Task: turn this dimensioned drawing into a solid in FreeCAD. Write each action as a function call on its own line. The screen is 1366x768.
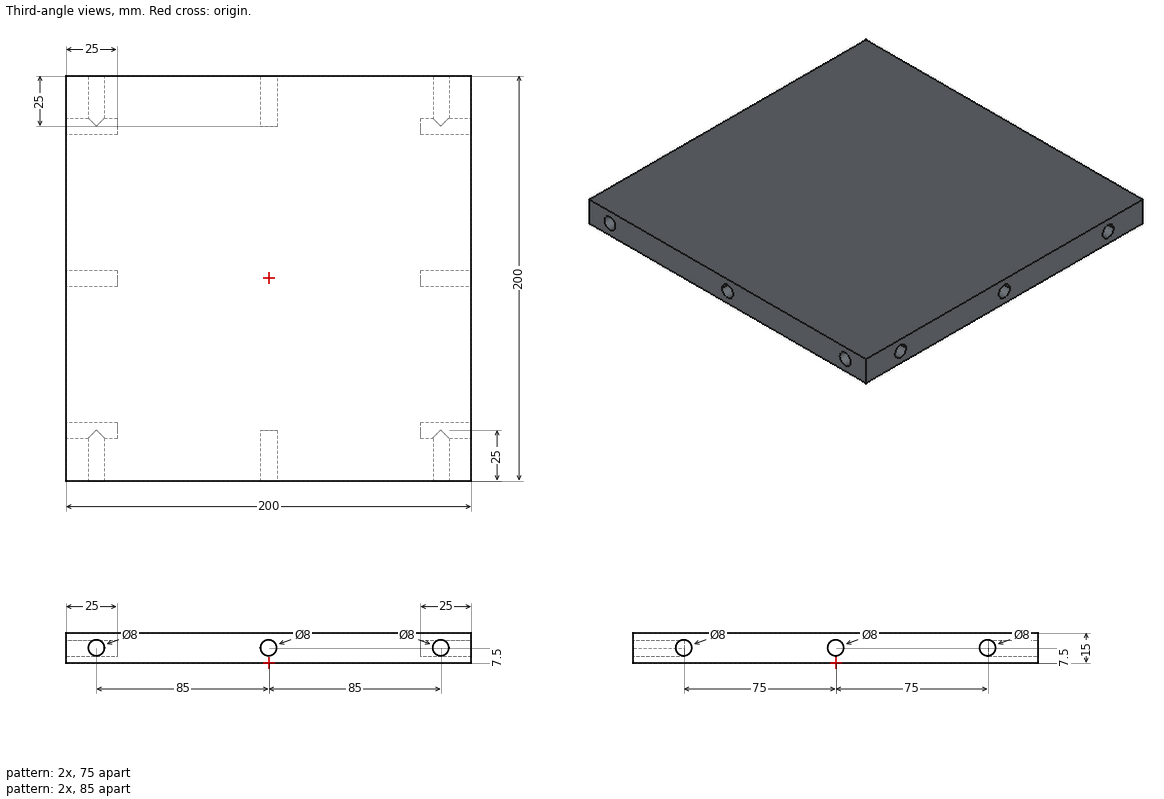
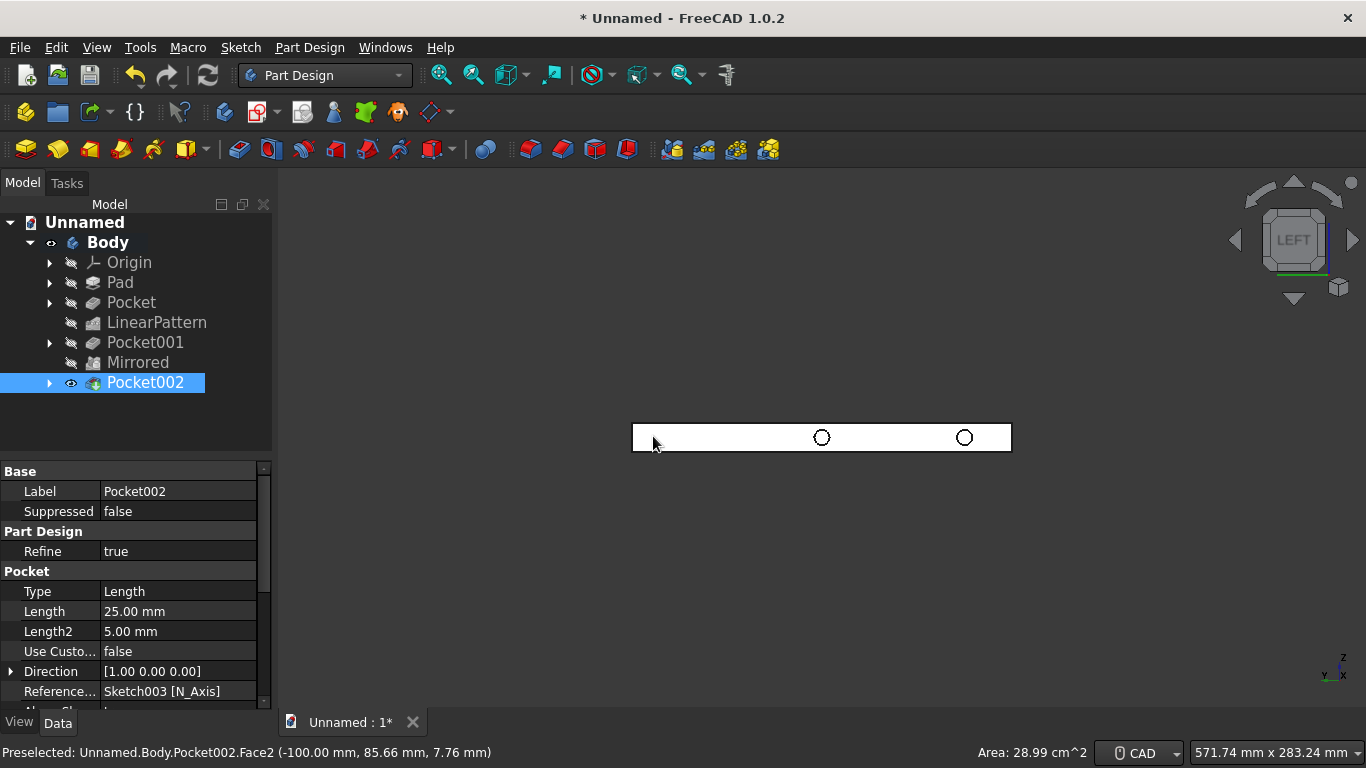
click(258, 112)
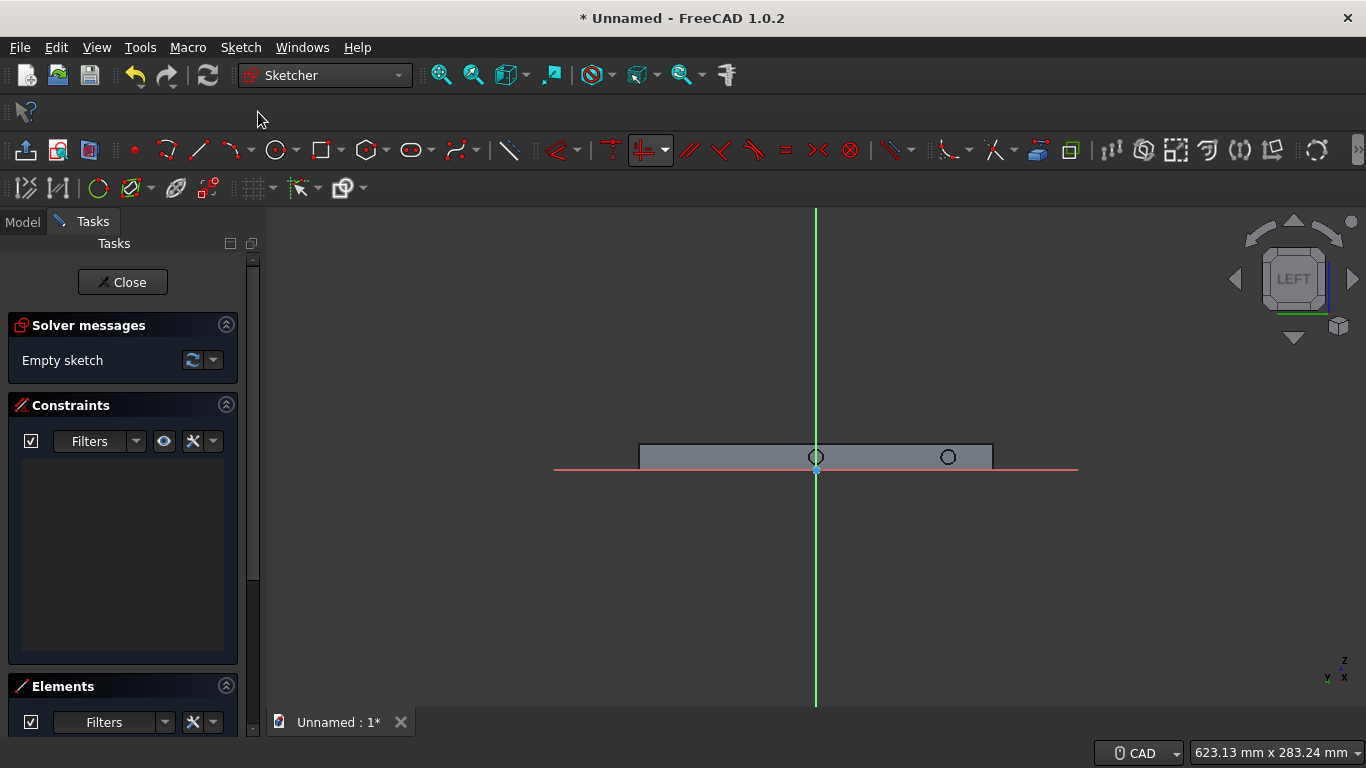
scroll(680, 457, up, 15)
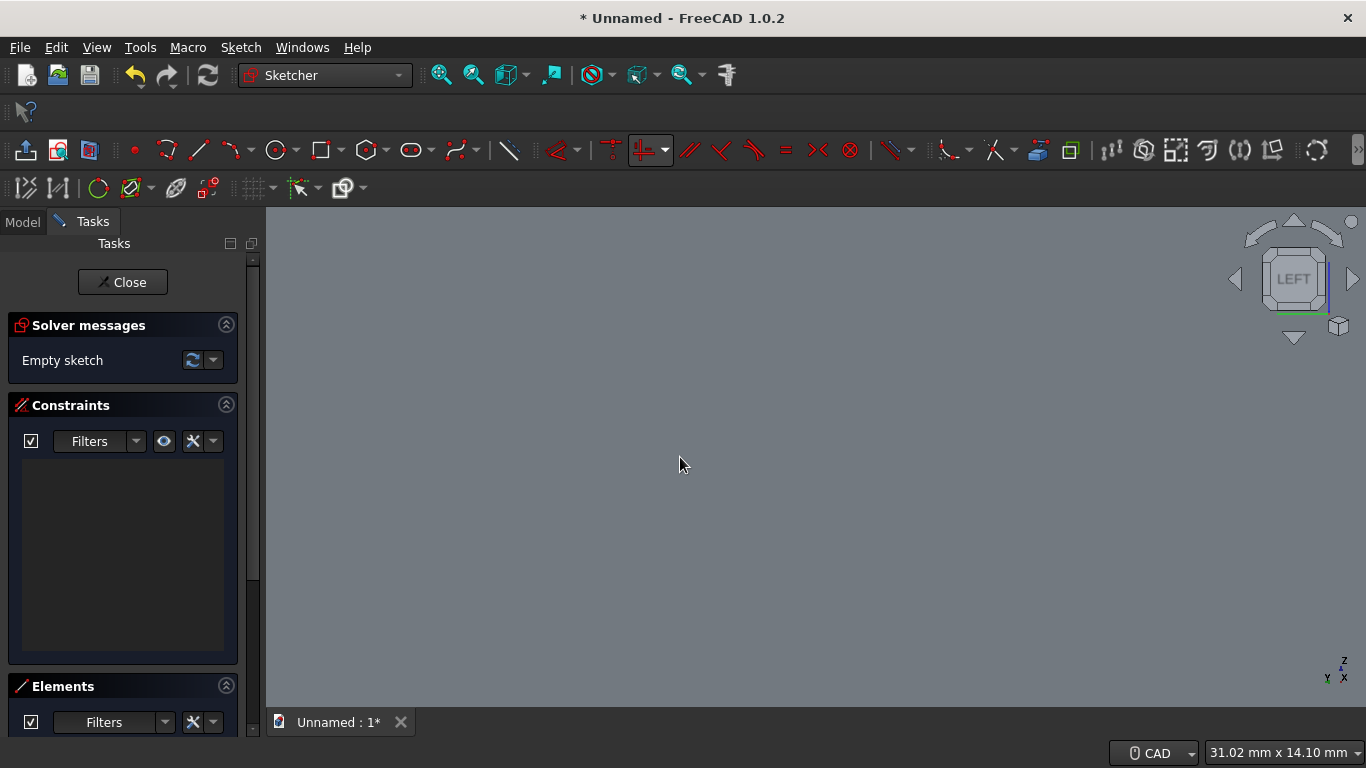
click(276, 150)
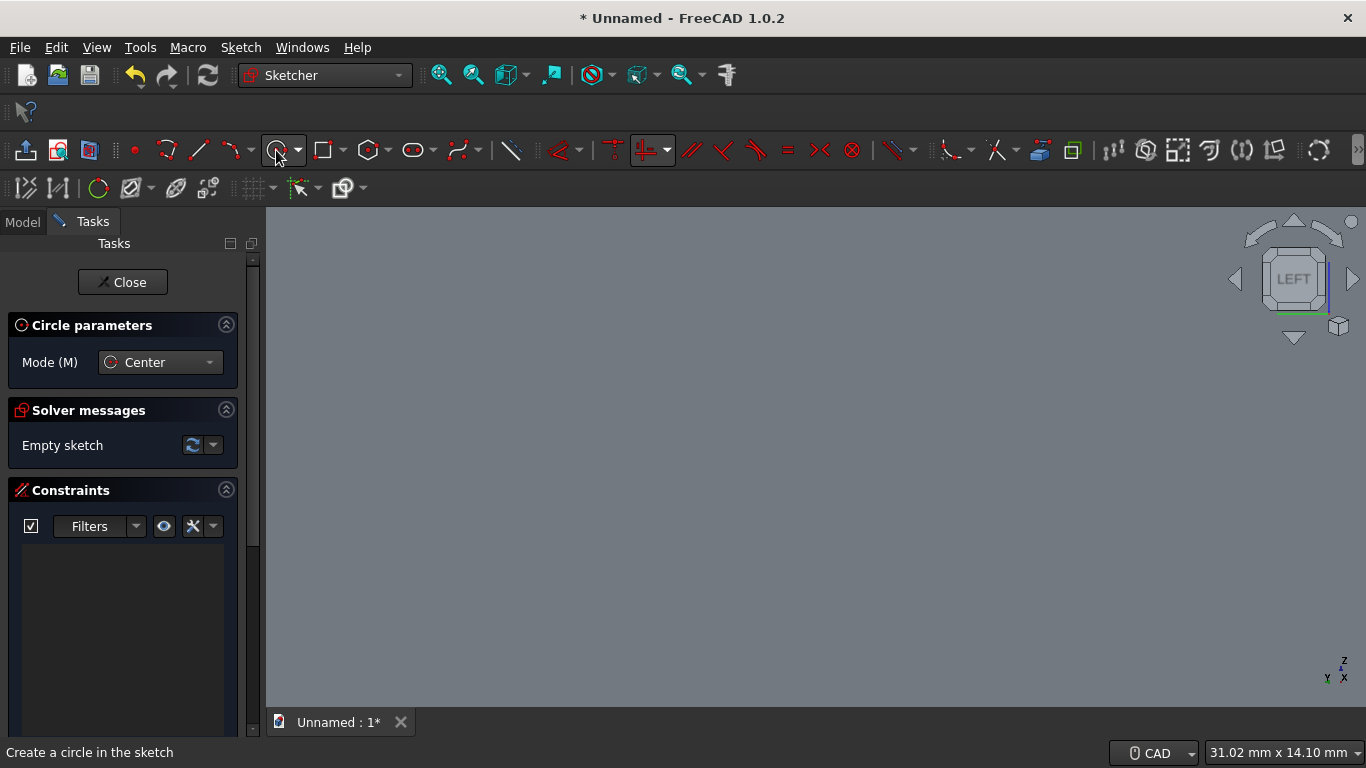
click(745, 447)
move(845, 347)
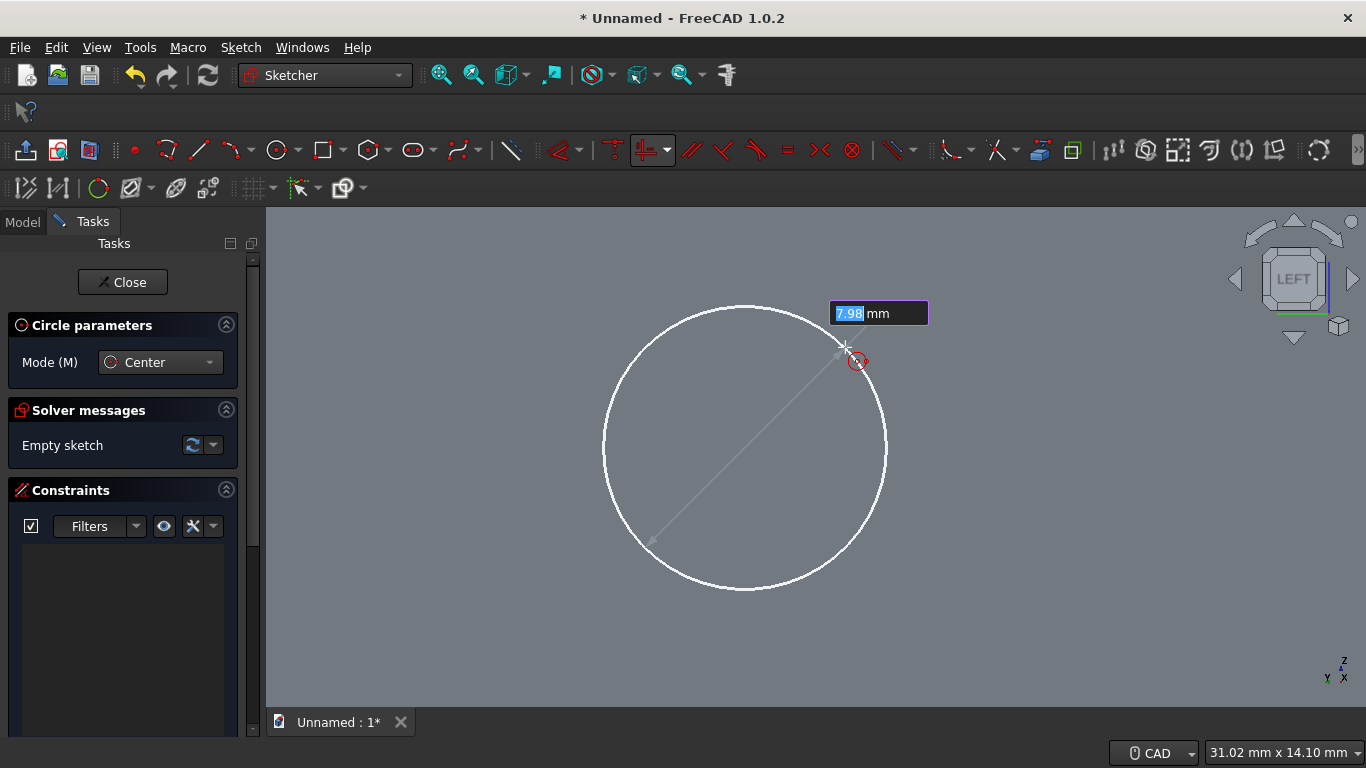
text(8)
key(Return)
key(Escape)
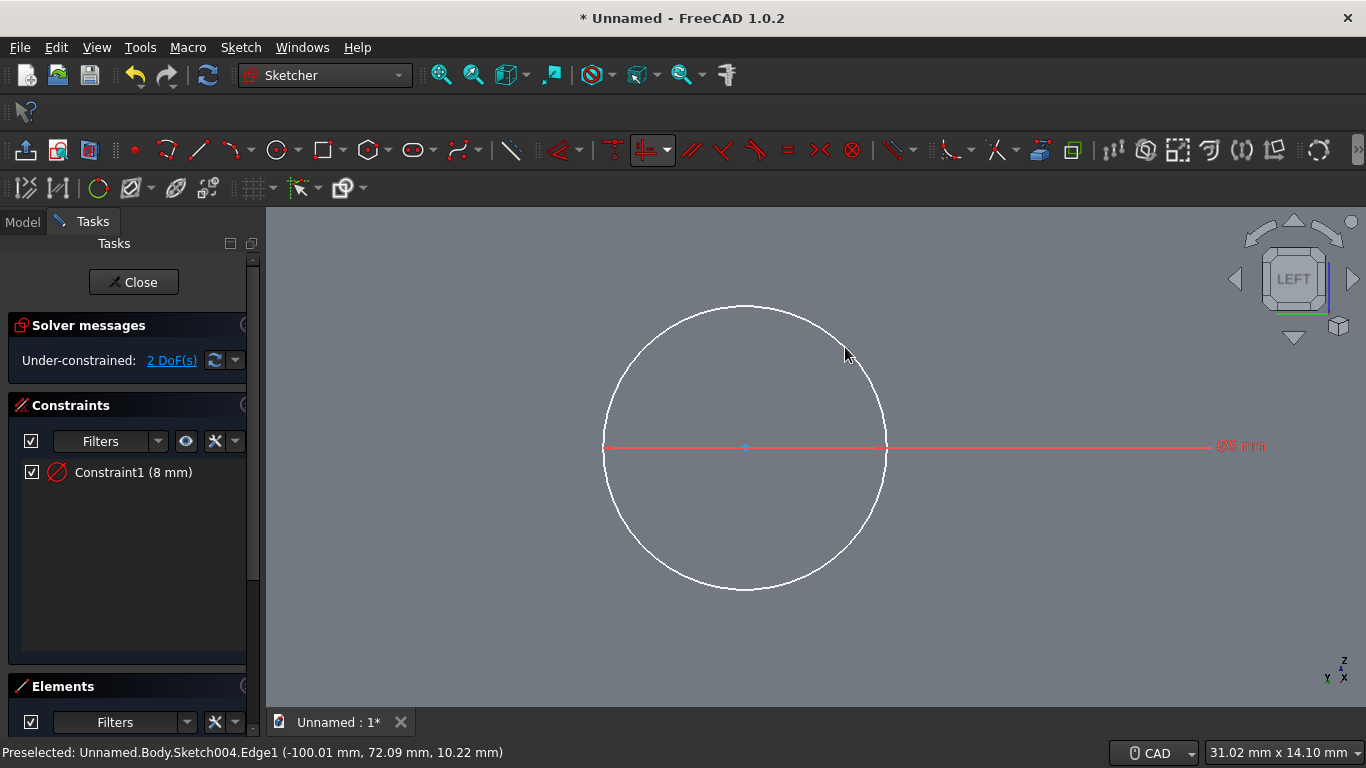
key(d)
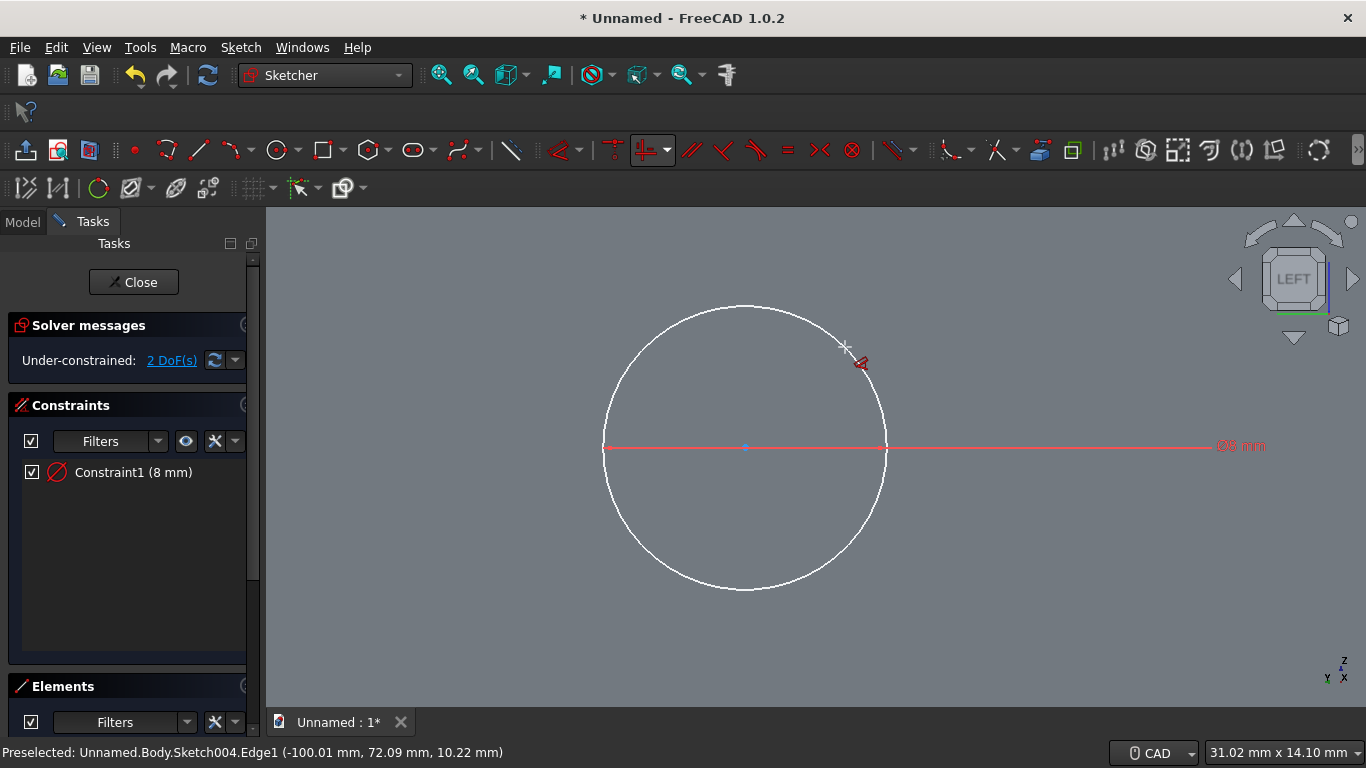
click(745, 448)
click(973, 414)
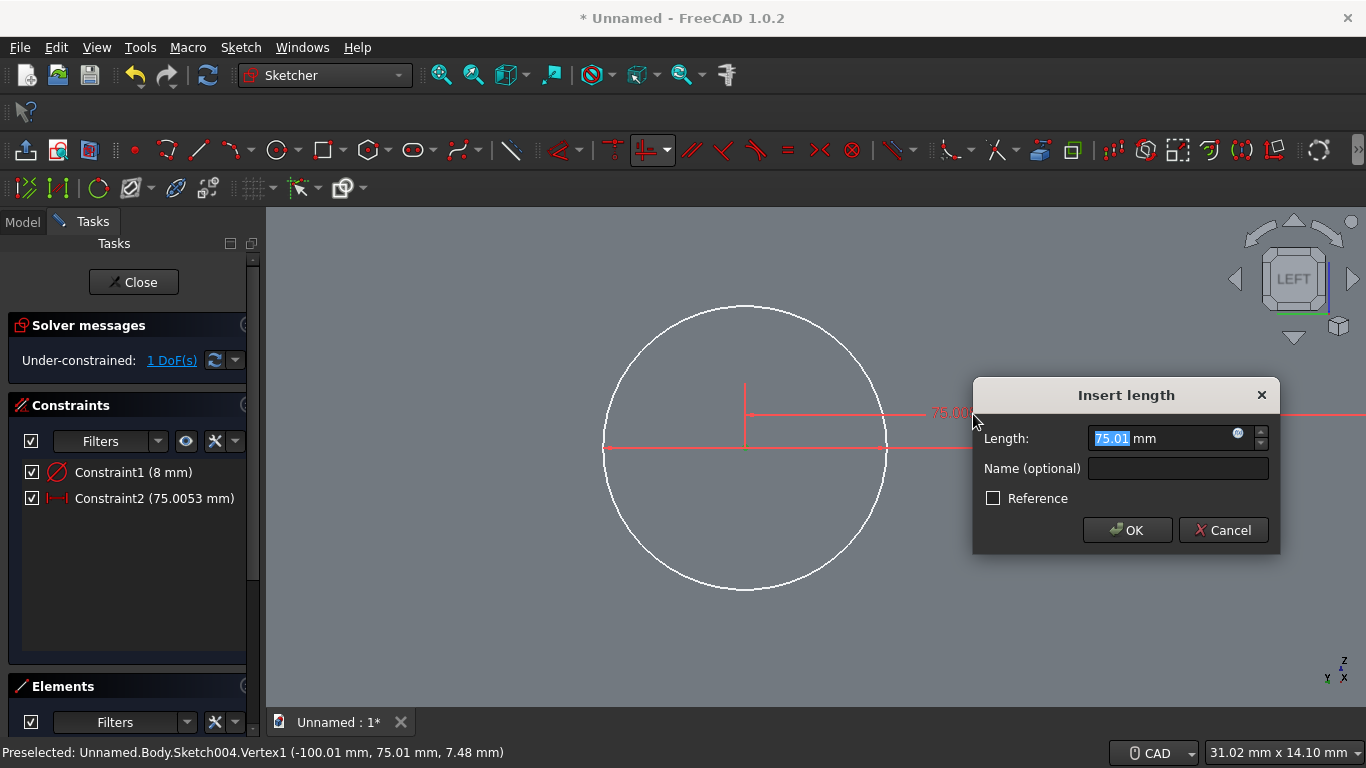
text(75)
key(Return)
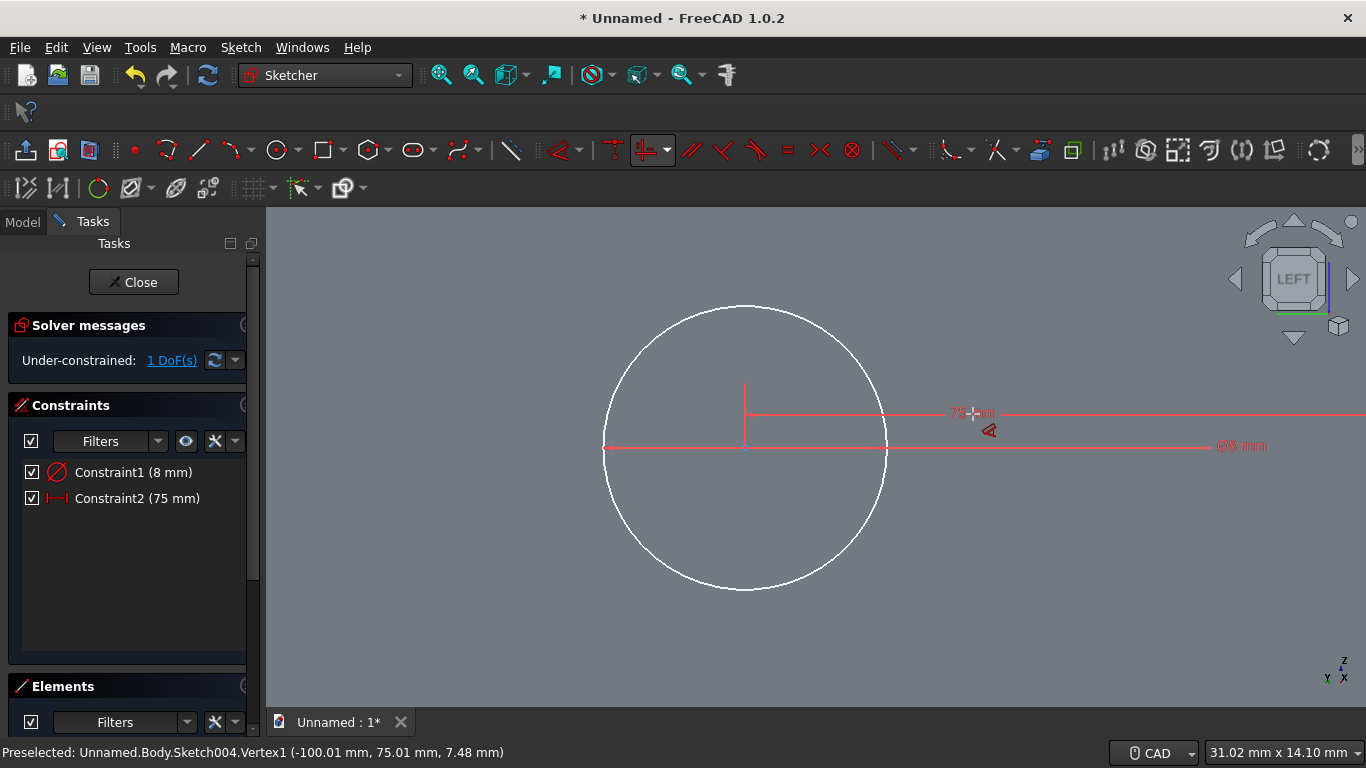
click(745, 448)
click(711, 564)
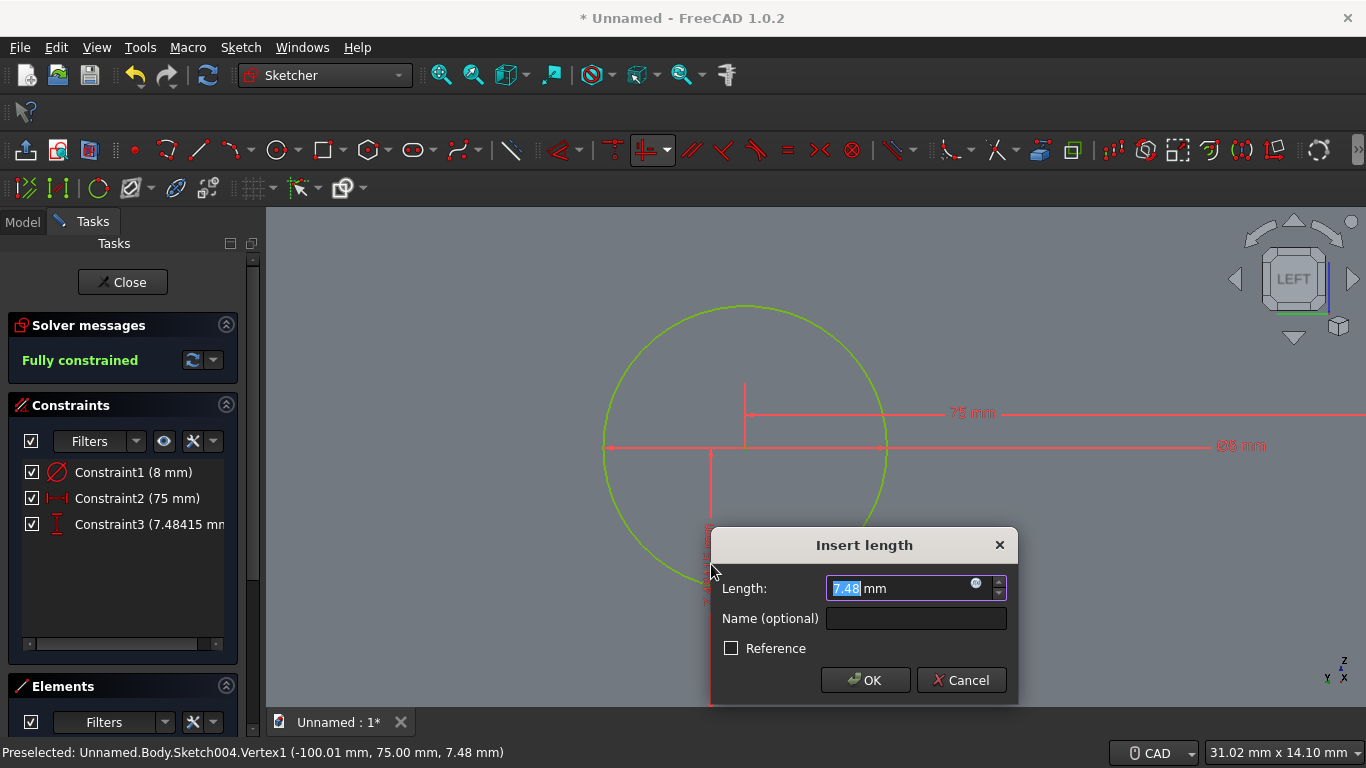
text(7.5)
key(Return)
key(Escape)